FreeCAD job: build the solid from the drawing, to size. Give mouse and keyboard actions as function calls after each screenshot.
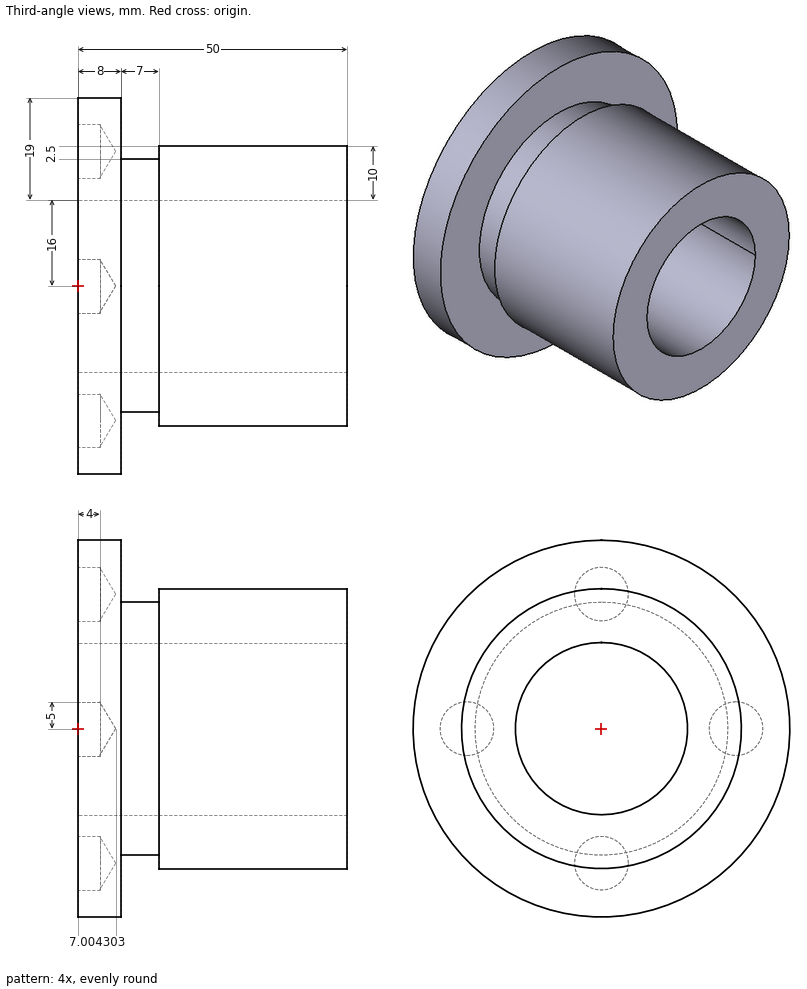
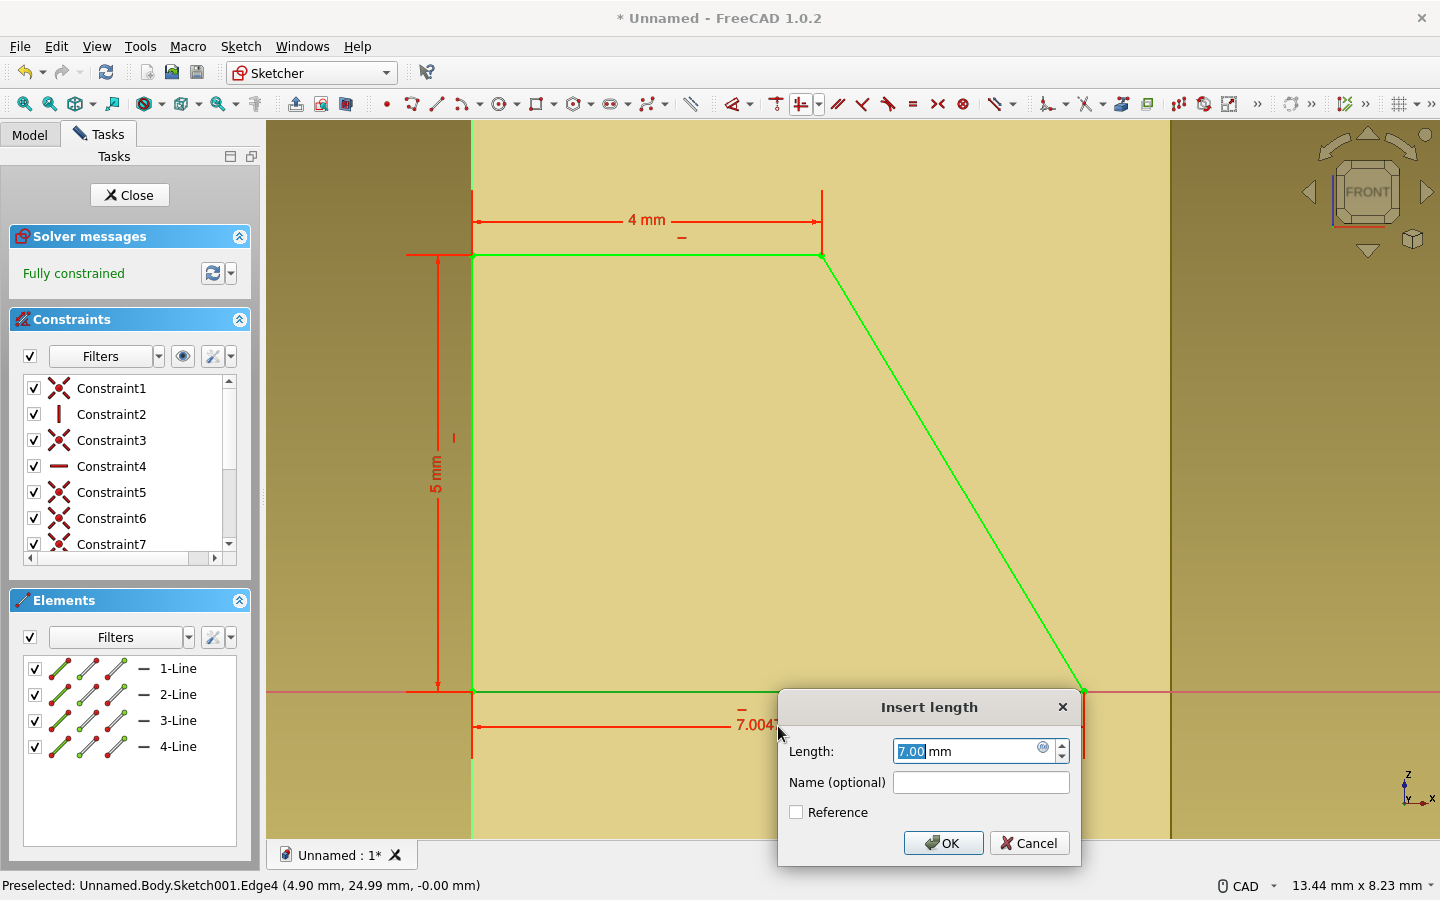
text(7.004303)
key(Return)
key(Escape)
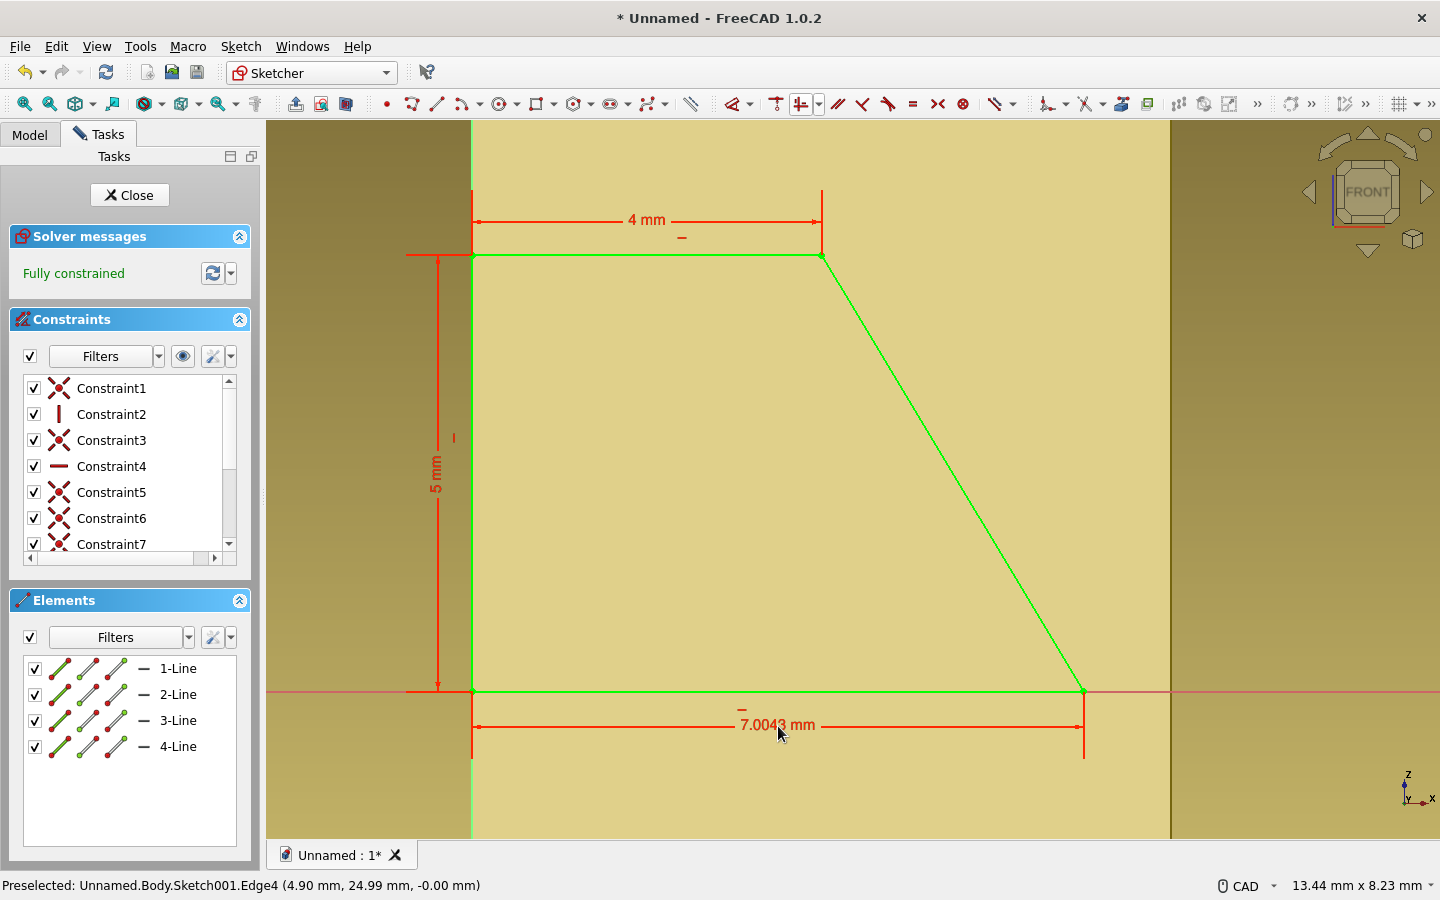
click(130, 195)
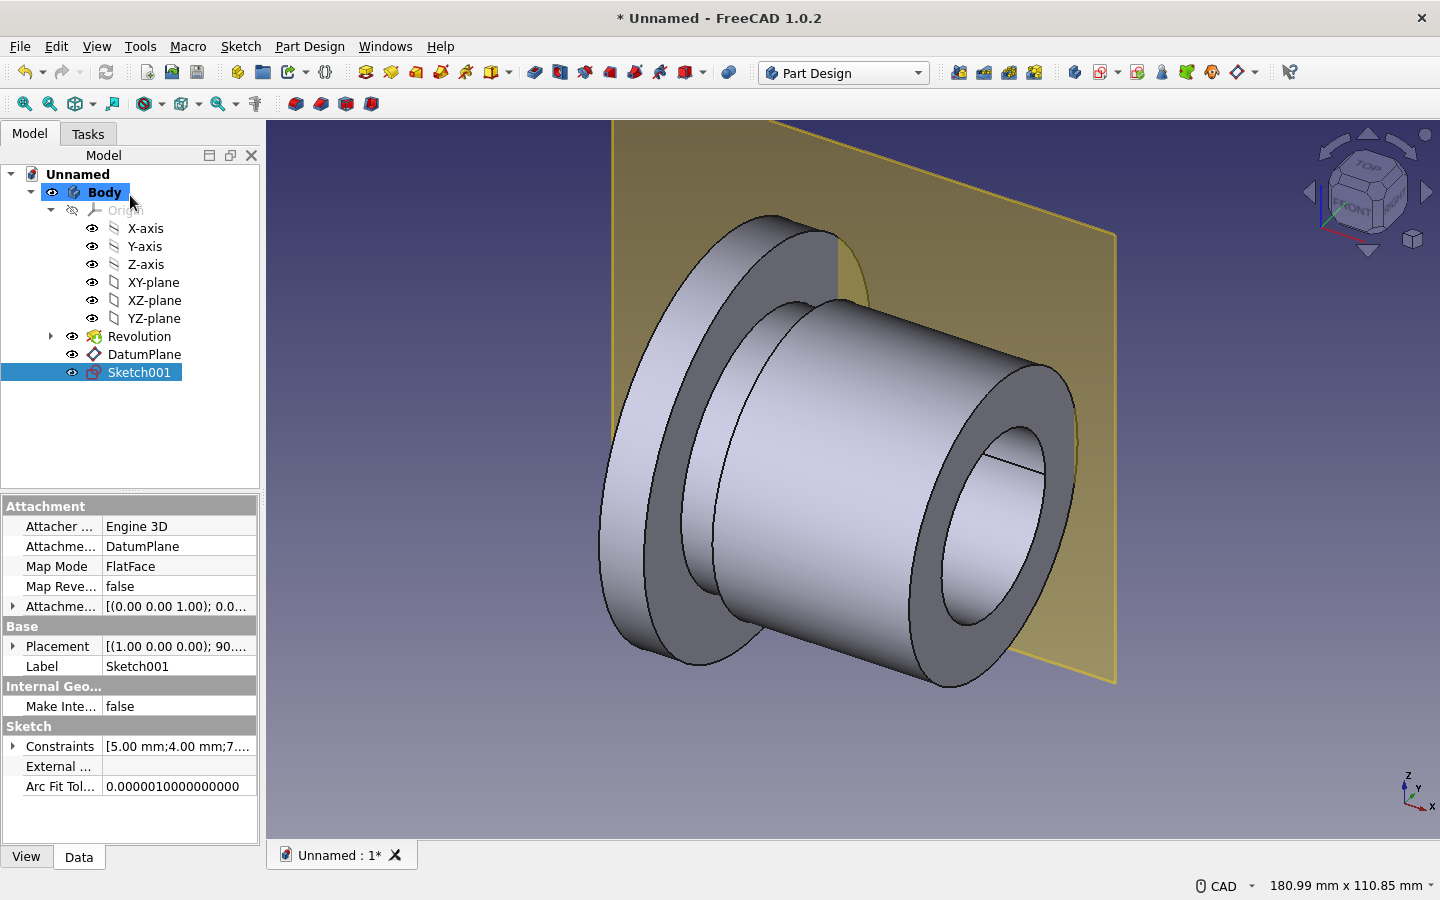
click(585, 72)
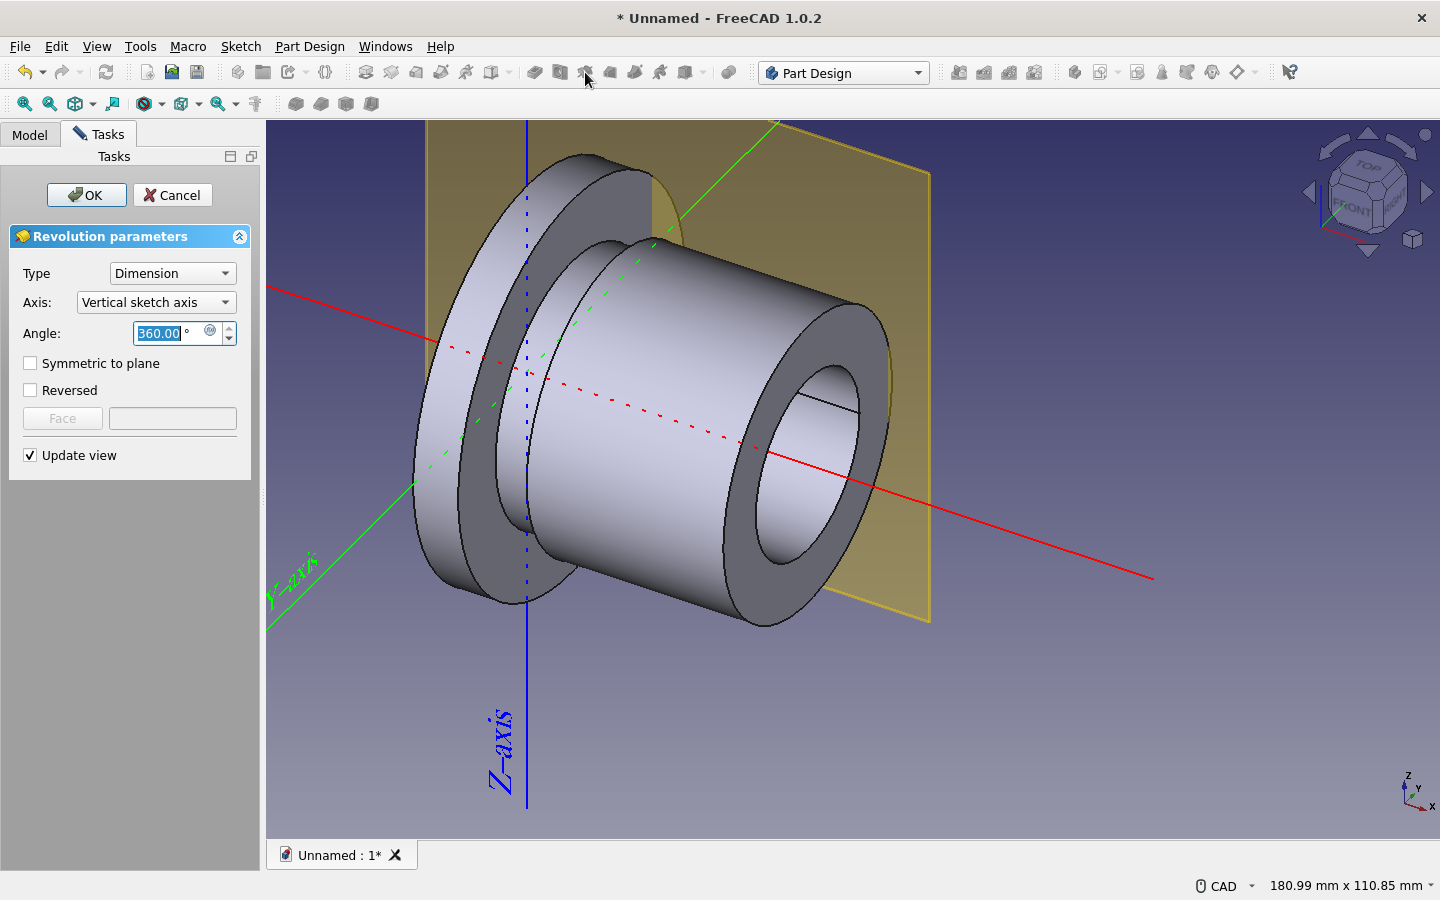
click(157, 302)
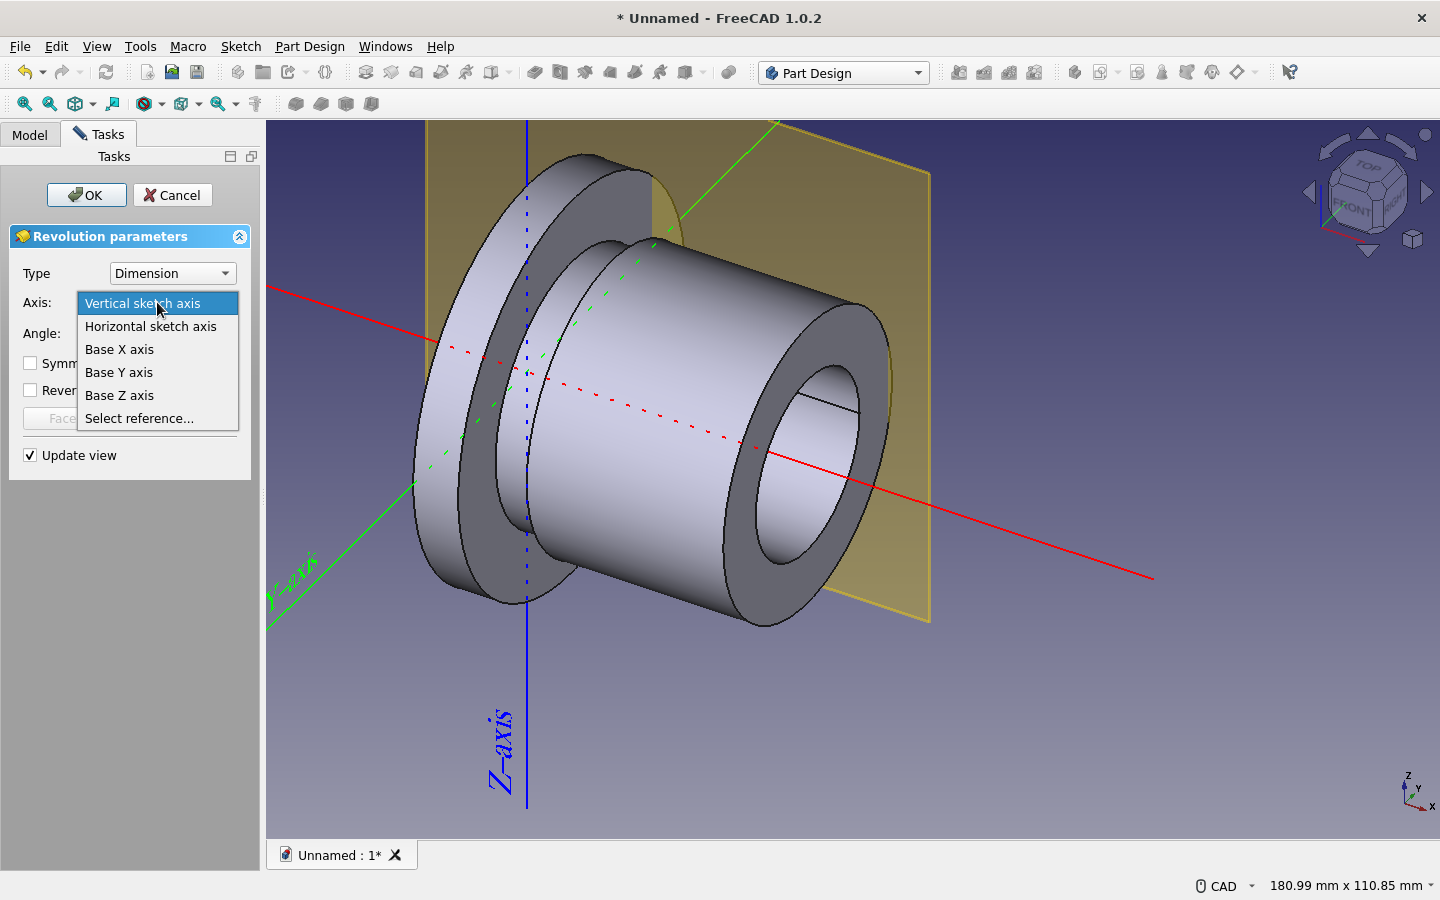
click(156, 326)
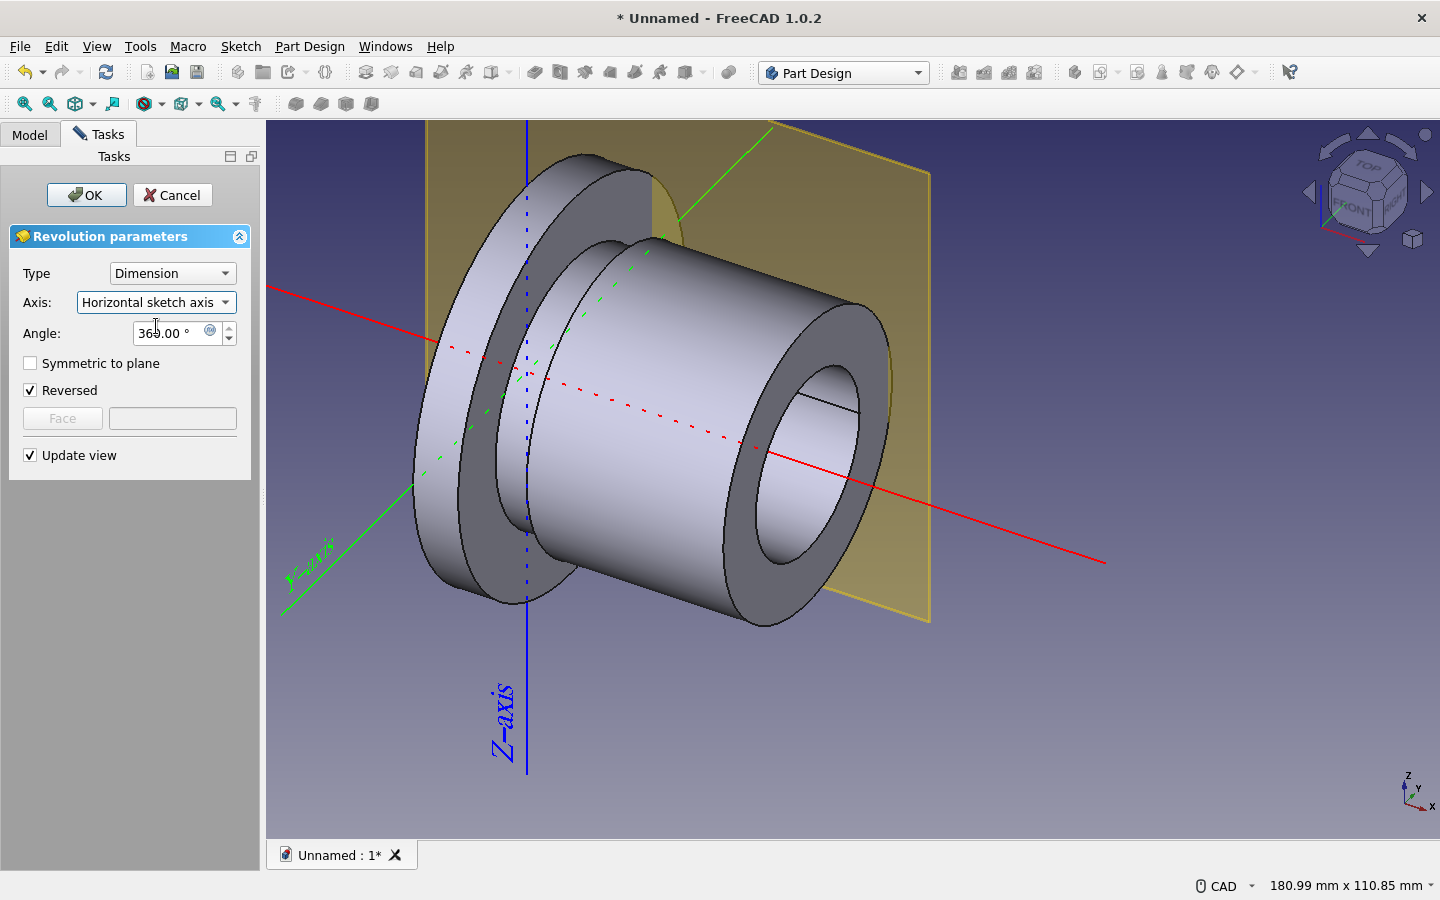
click(87, 195)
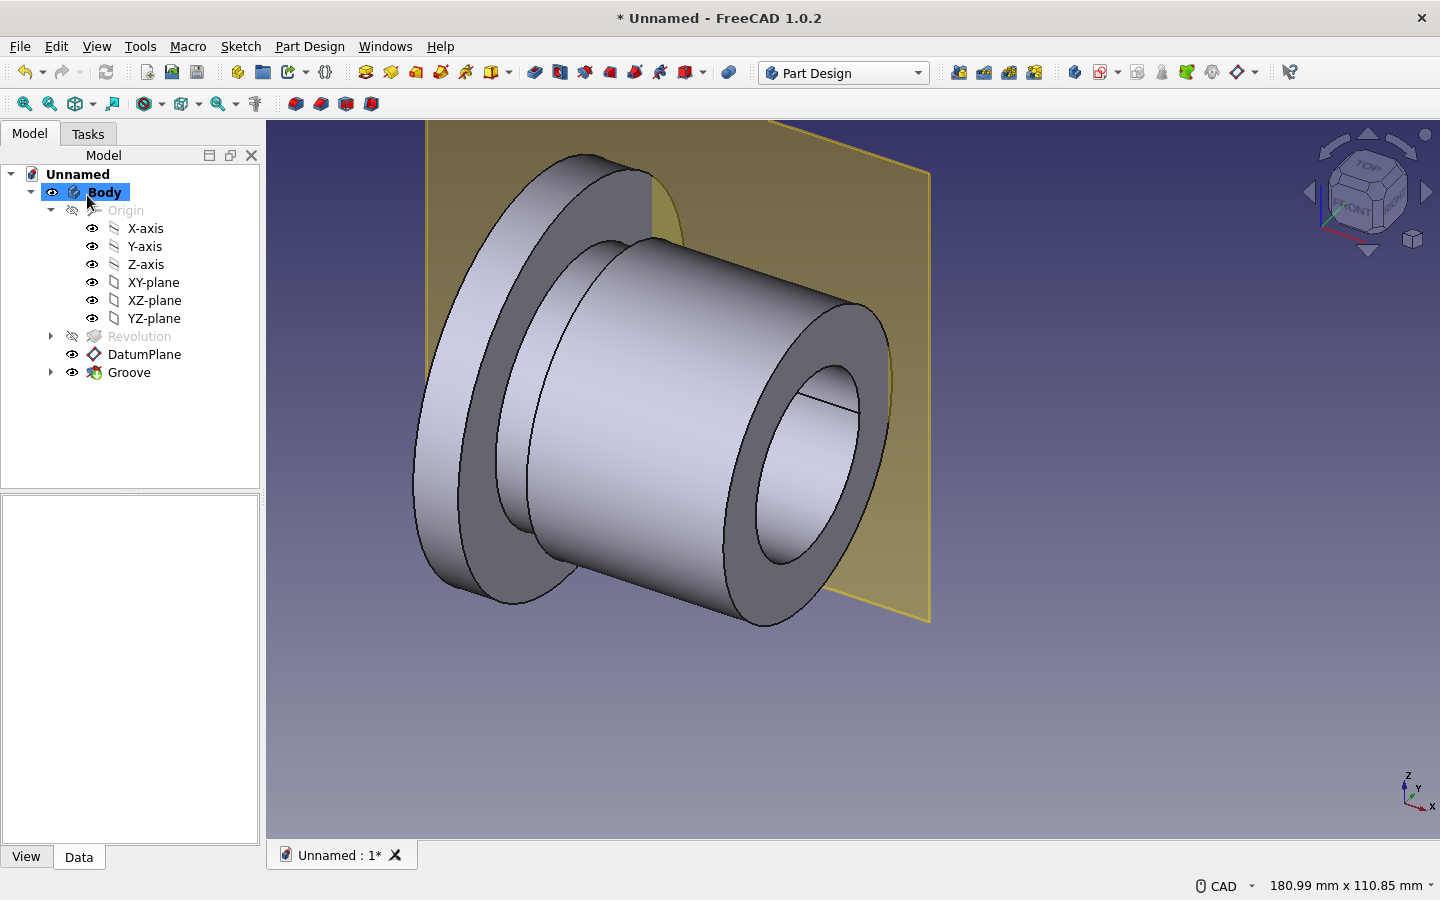
click(117, 354)
key(space)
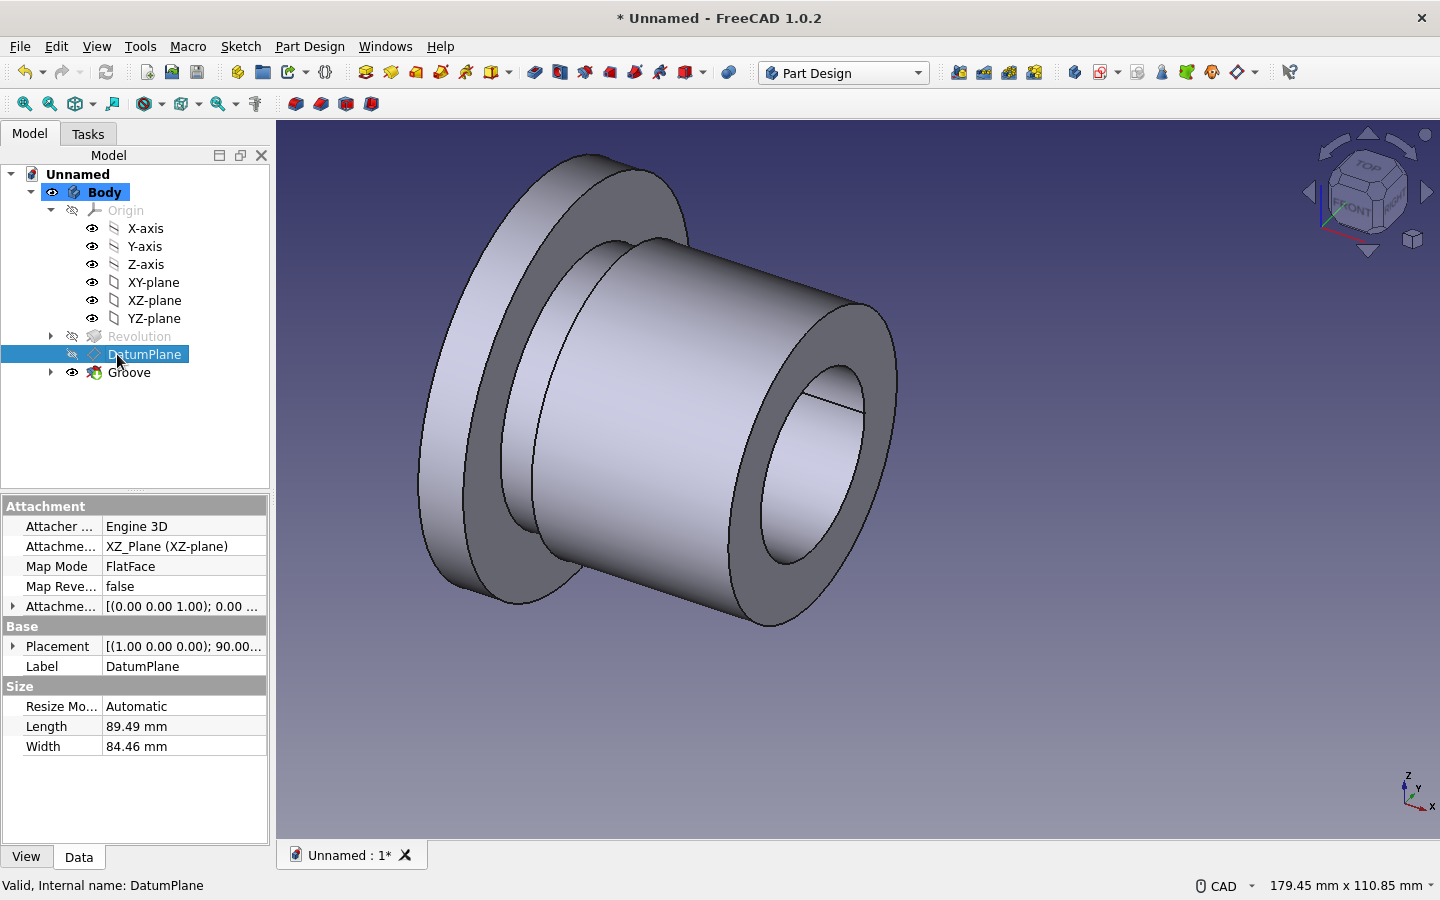
click(25, 104)